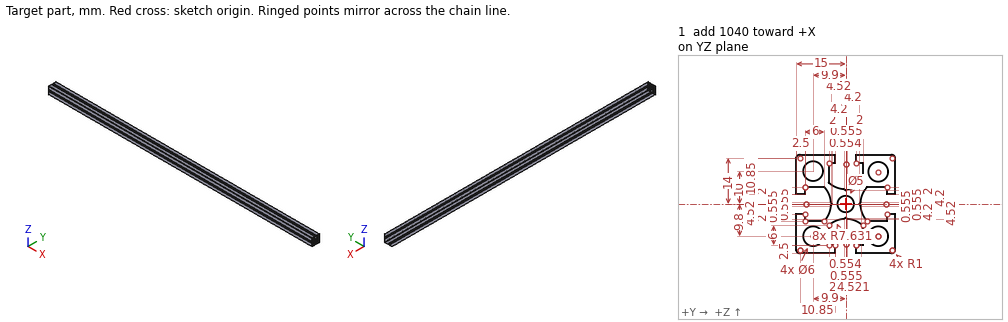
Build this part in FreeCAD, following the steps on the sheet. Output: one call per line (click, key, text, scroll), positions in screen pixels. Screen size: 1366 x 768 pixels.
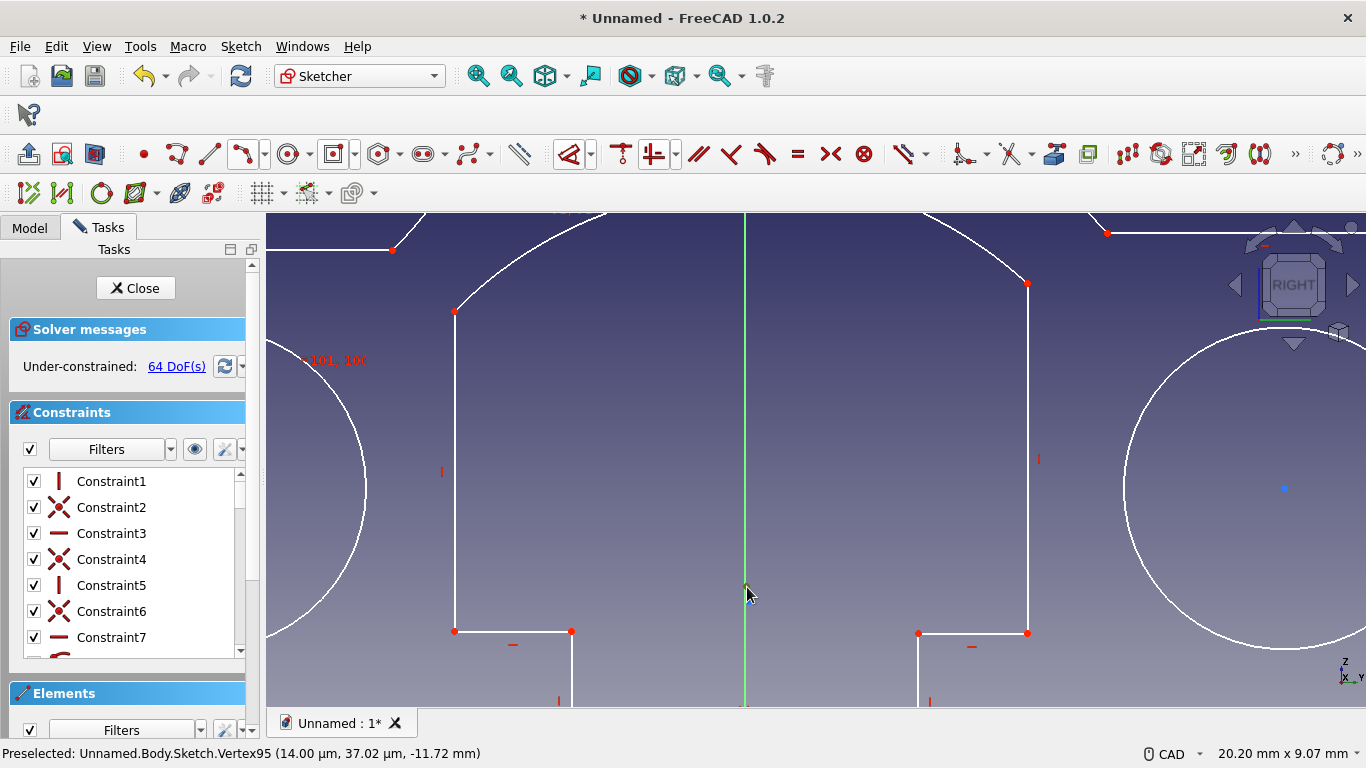
scroll(748, 589, down, 8)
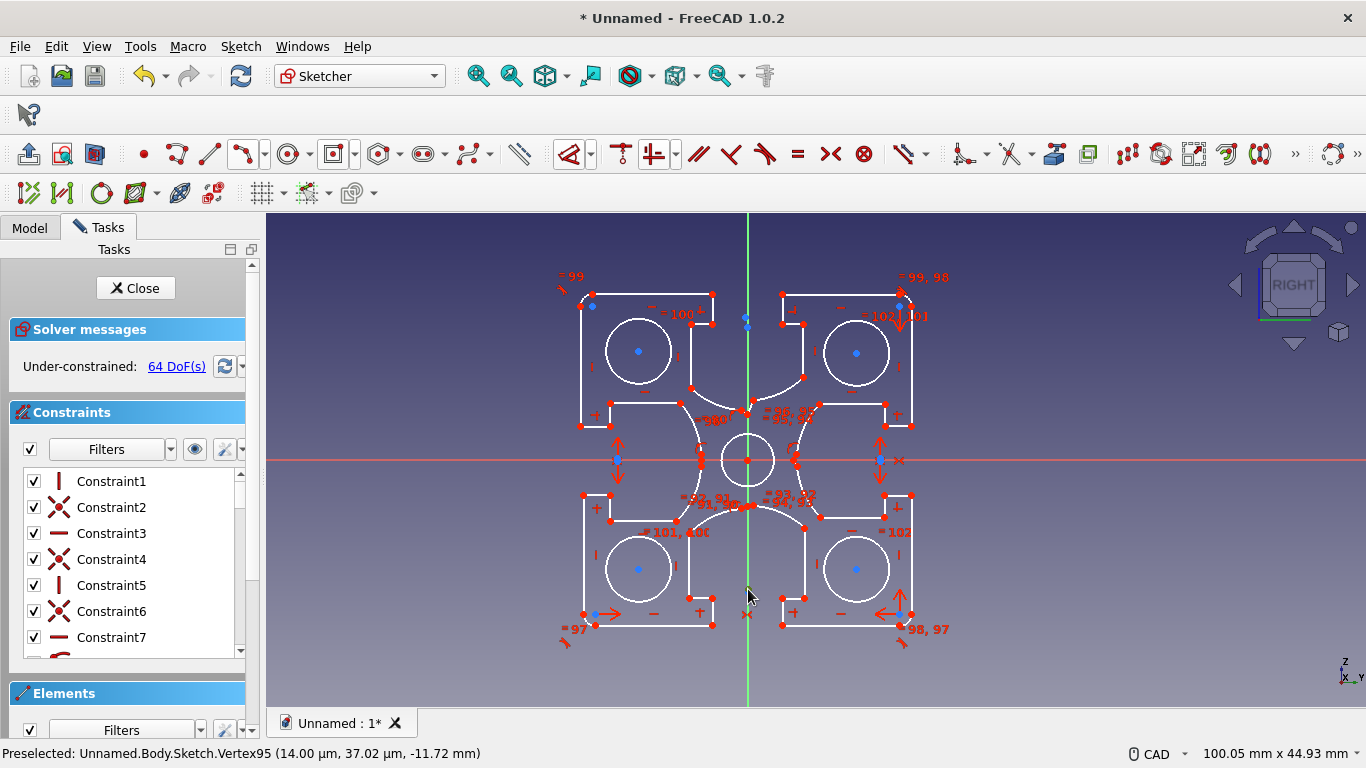
click(746, 317)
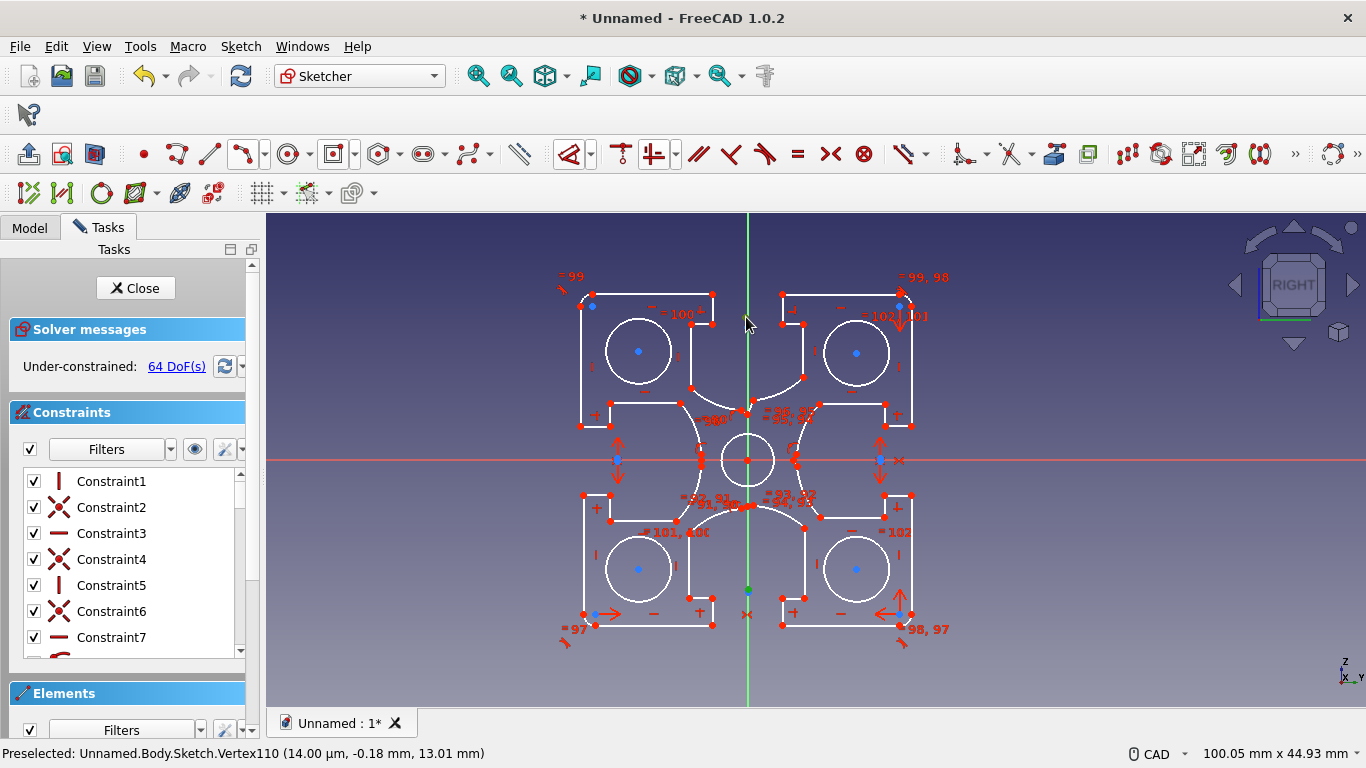
click(359, 460)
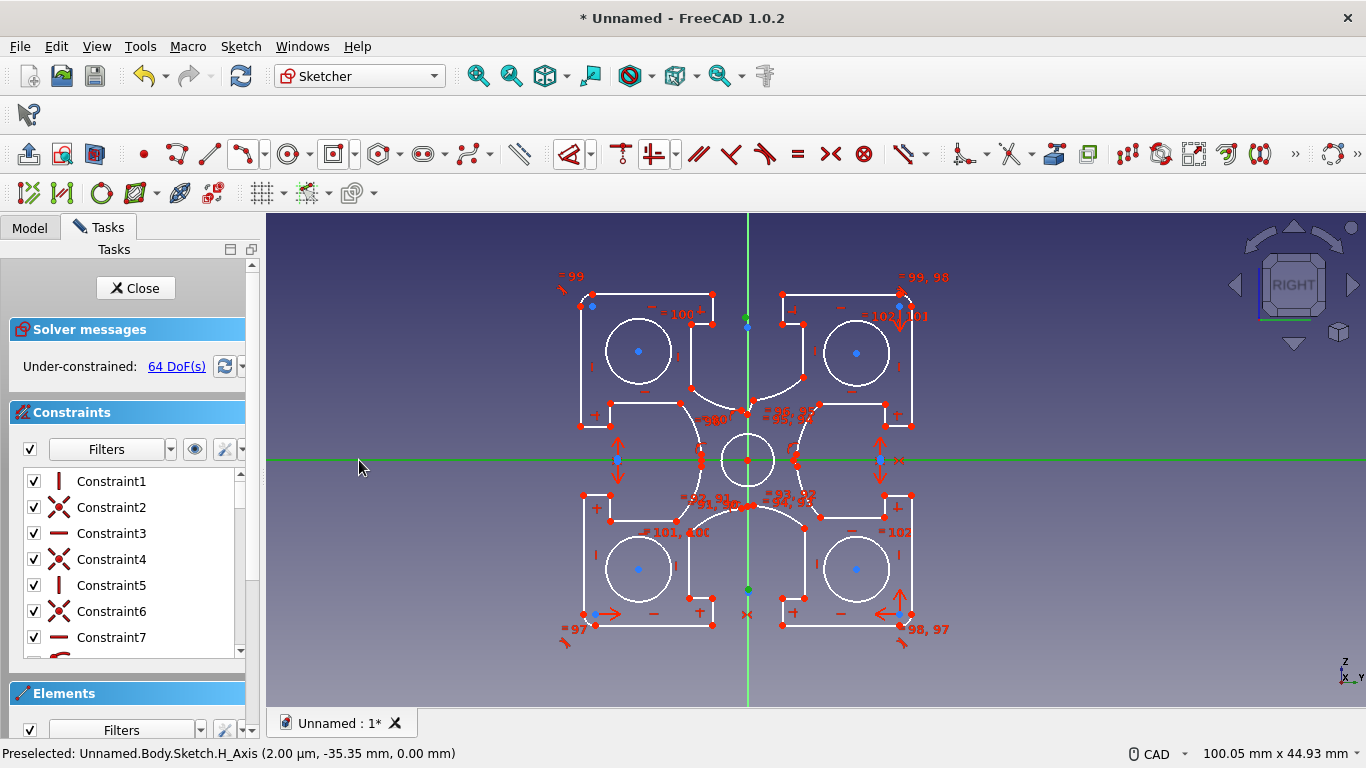
click(831, 154)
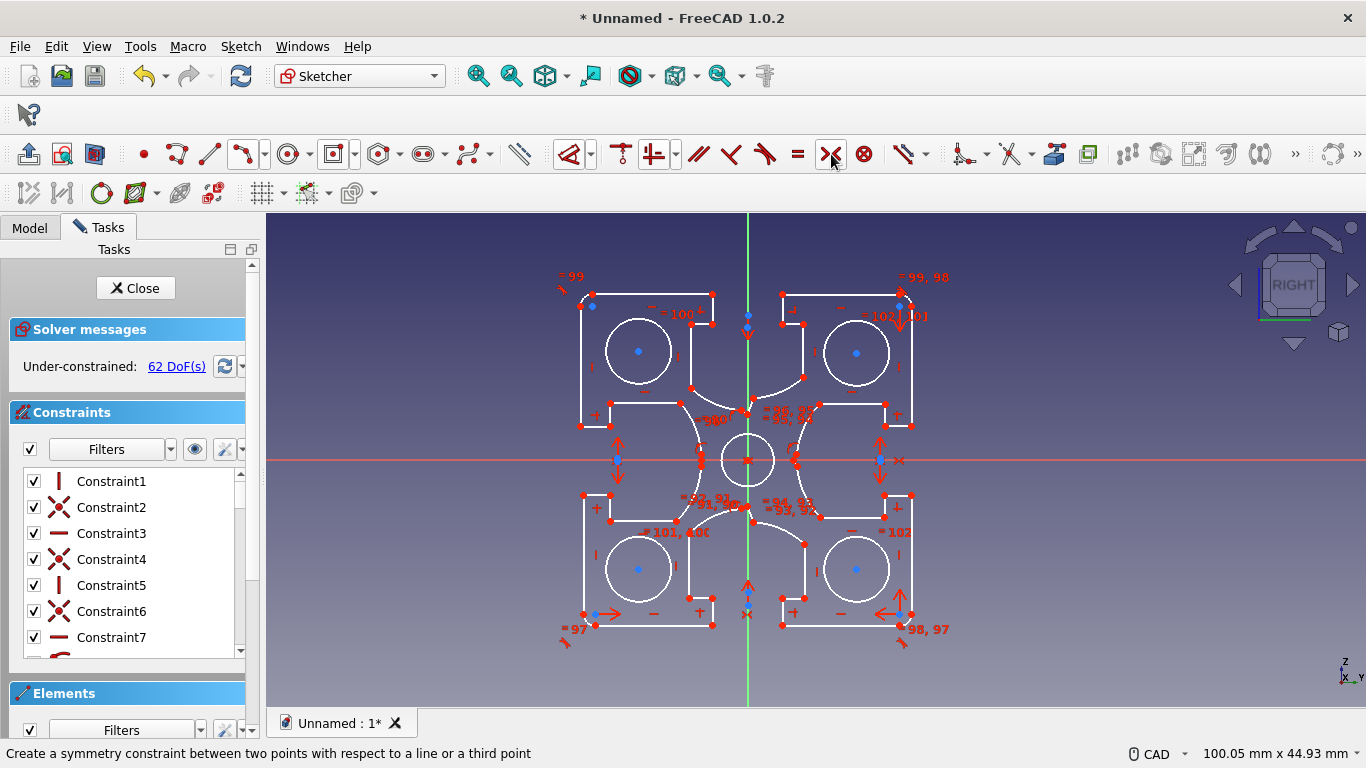
click(749, 592)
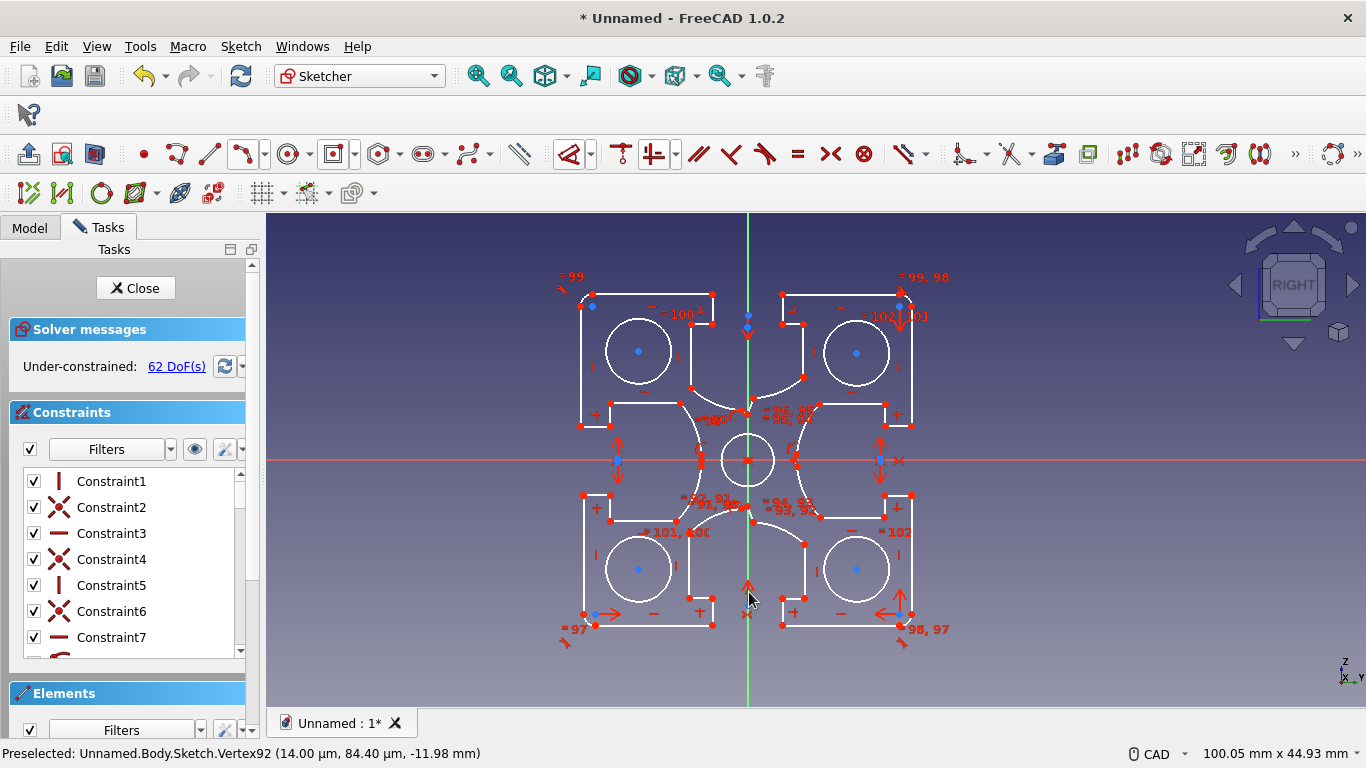
click(748, 327)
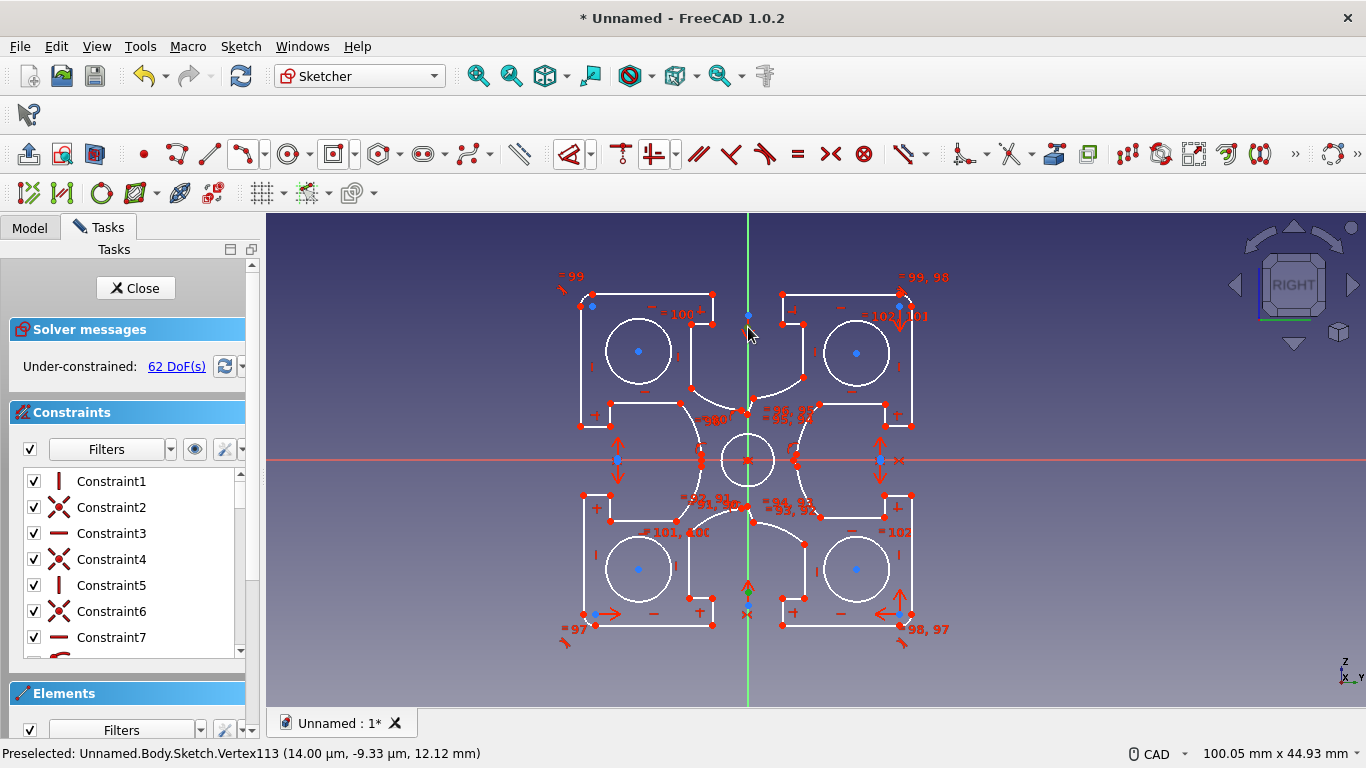
click(359, 460)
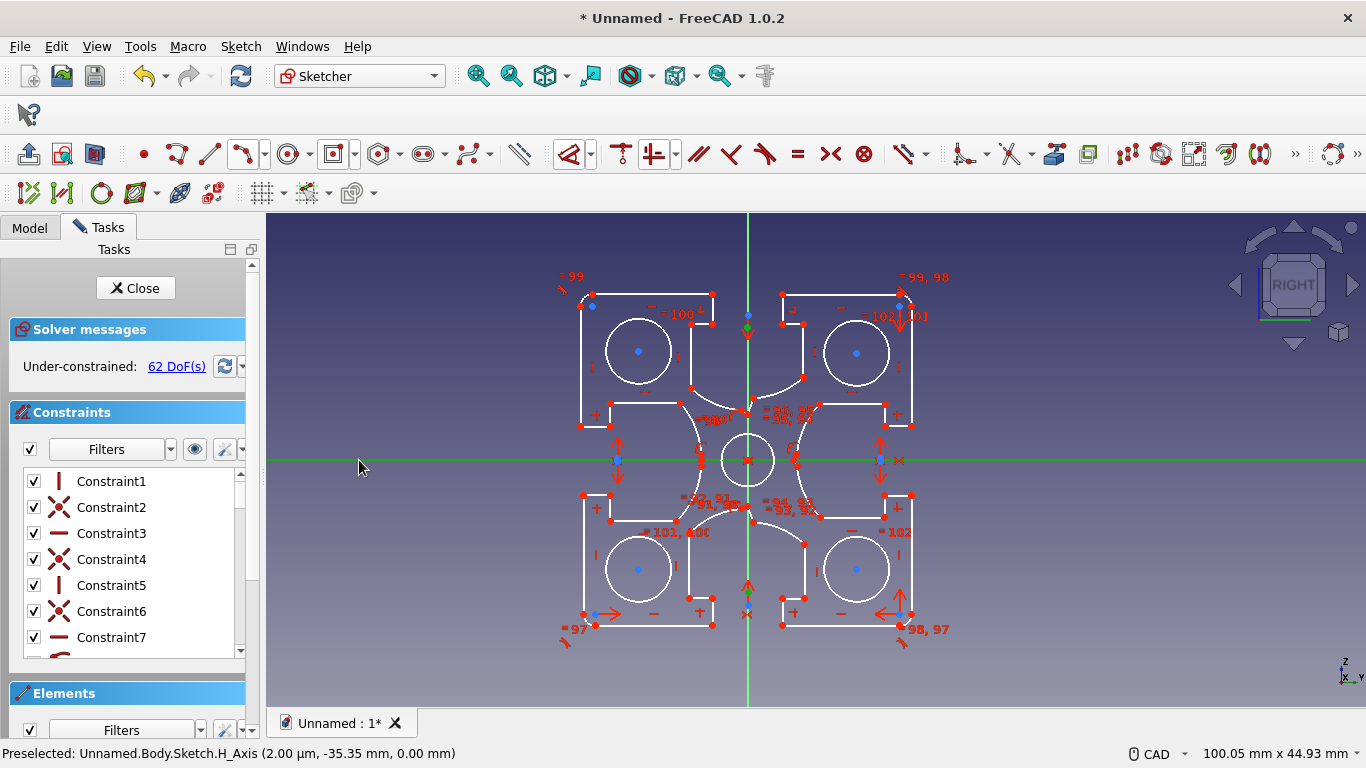
click(831, 154)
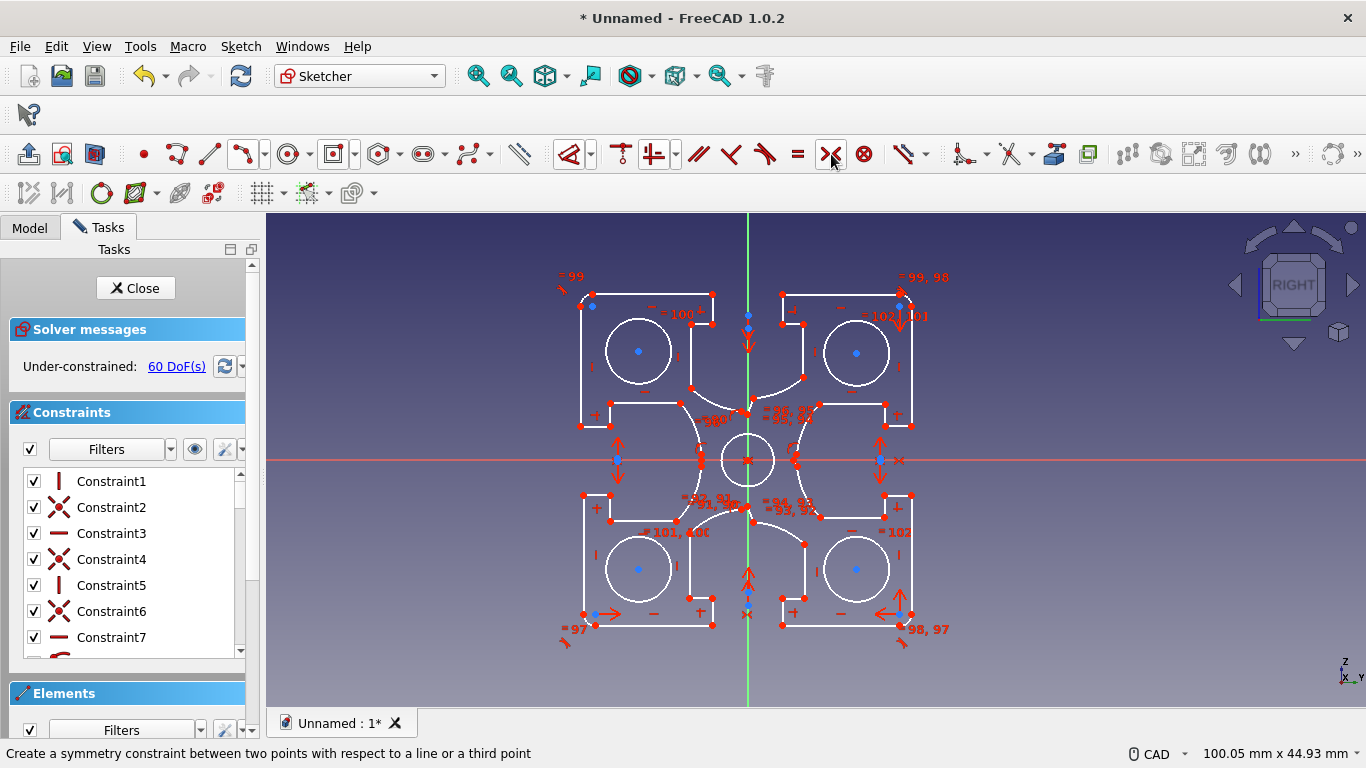
click(596, 614)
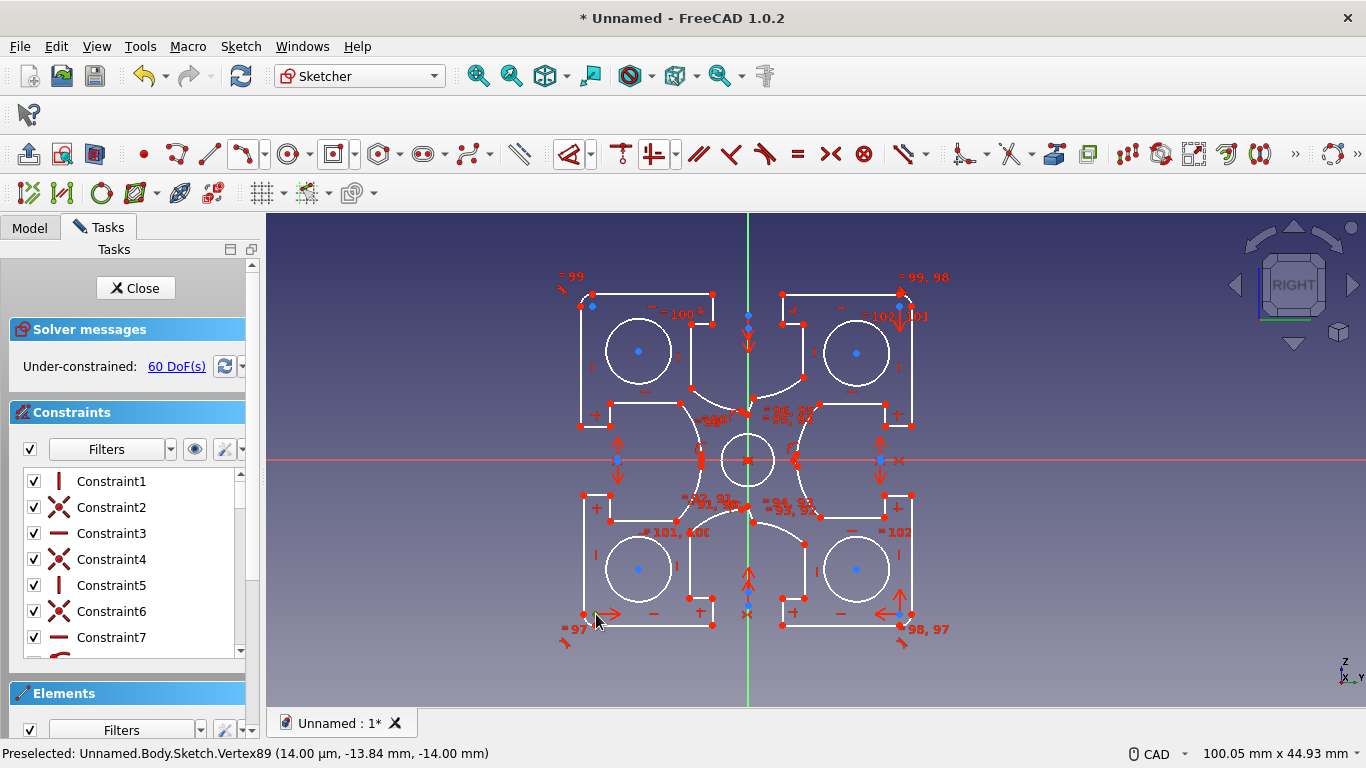
click(592, 306)